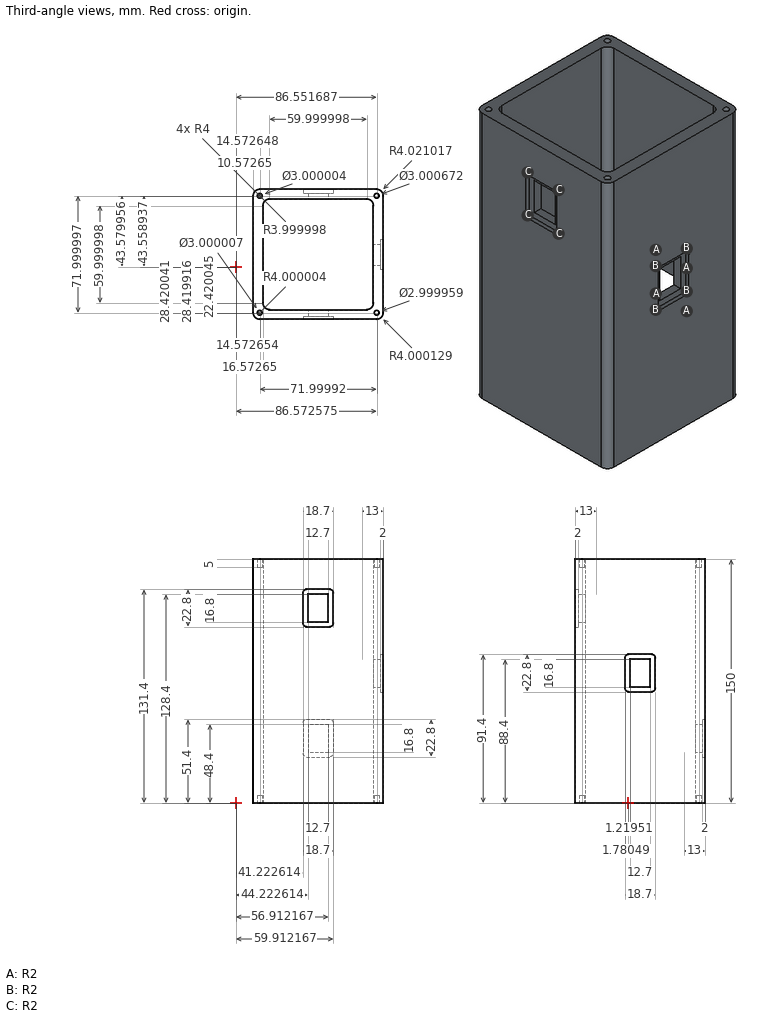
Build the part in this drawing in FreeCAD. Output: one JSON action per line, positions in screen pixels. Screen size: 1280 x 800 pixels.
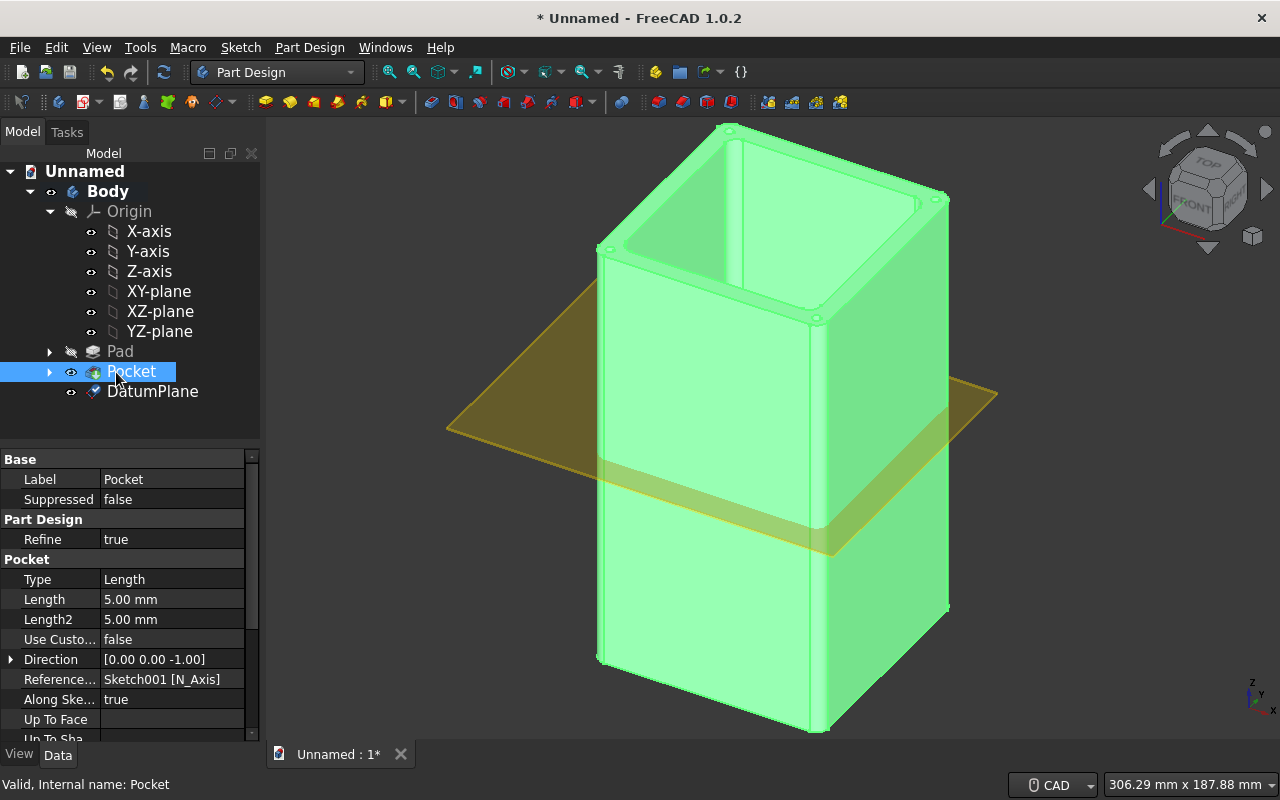
{"action": "left_click", "coordinate": [768, 102]}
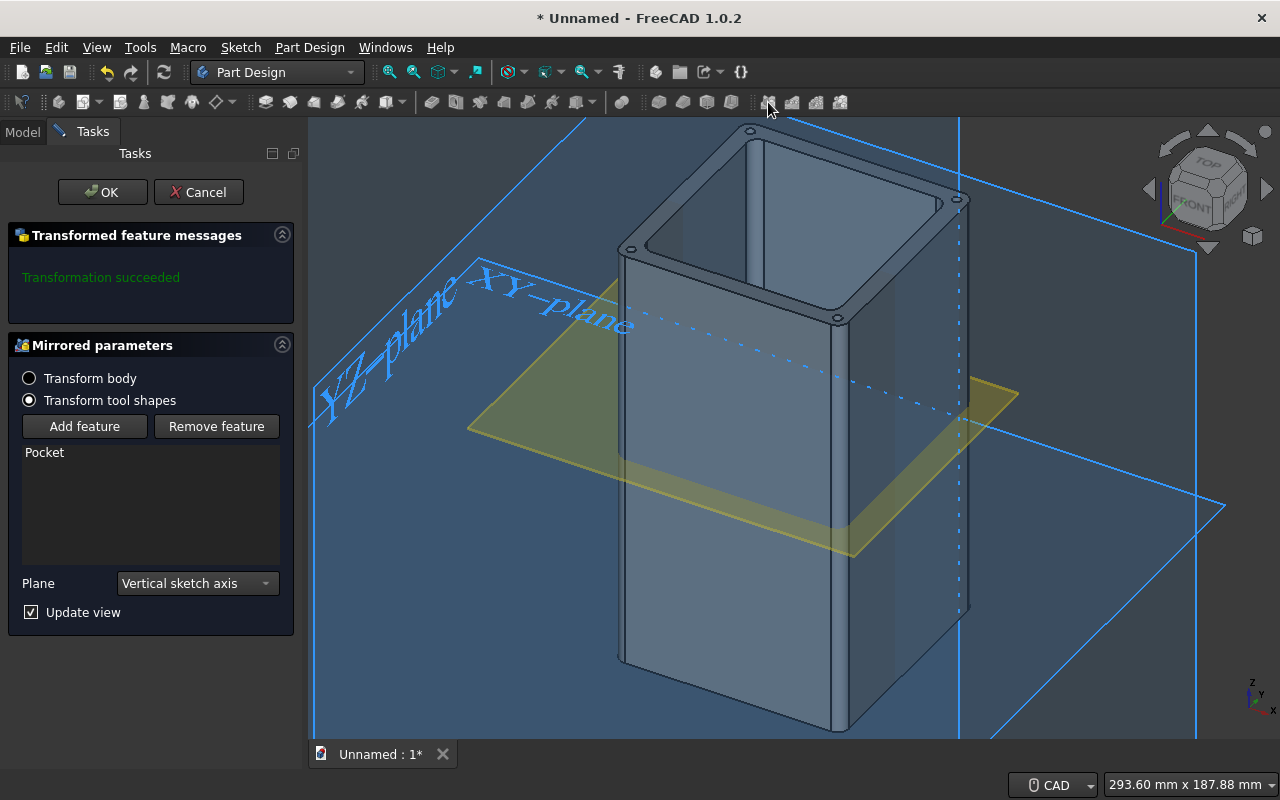
{"action": "left_click", "coordinate": [198, 584]}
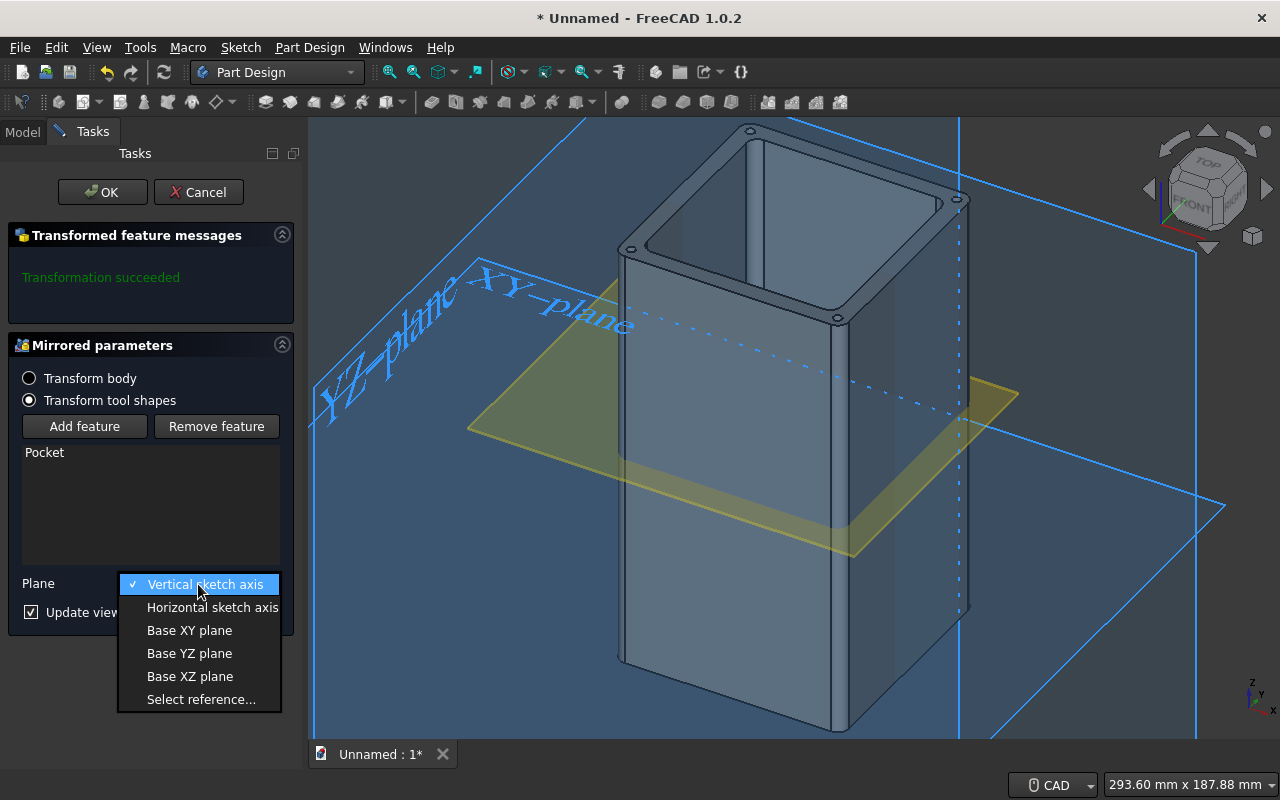
{"action": "left_click", "coordinate": [198, 700]}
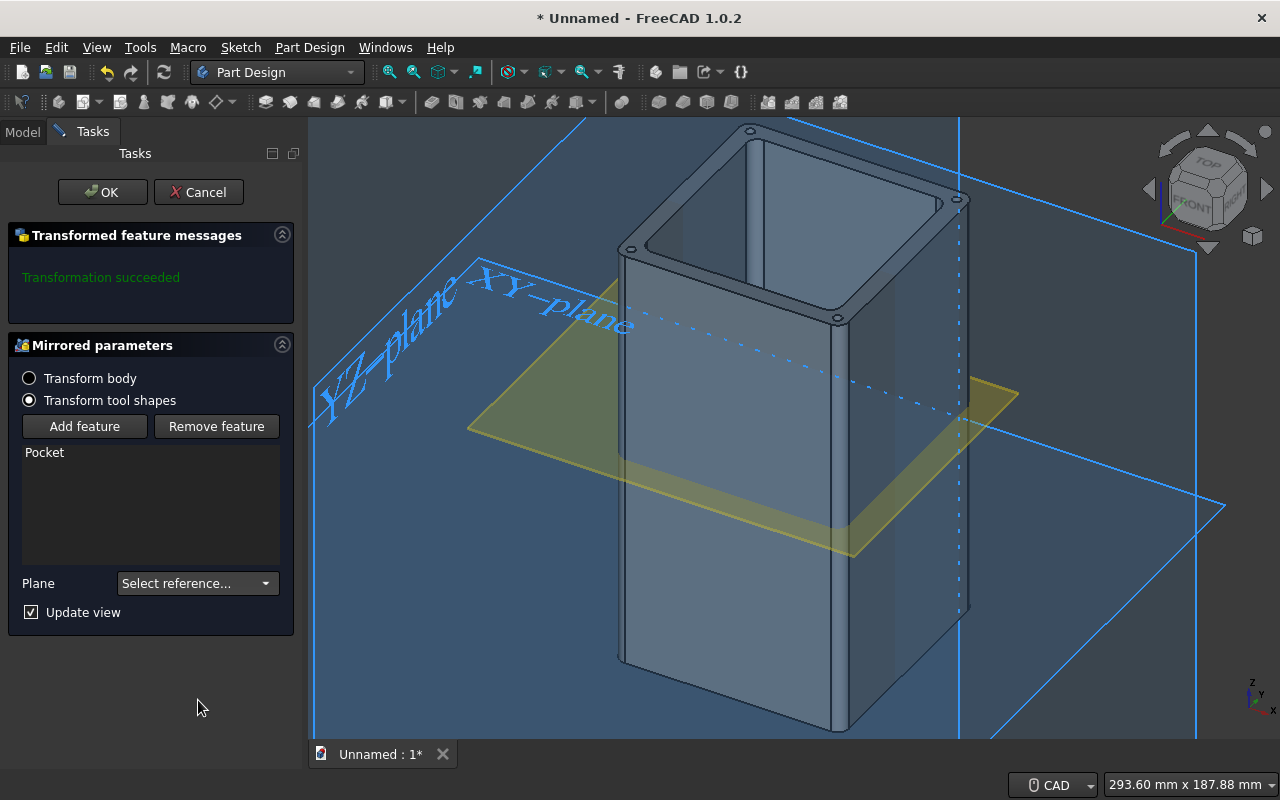
{"action": "left_click", "coordinate": [23, 131]}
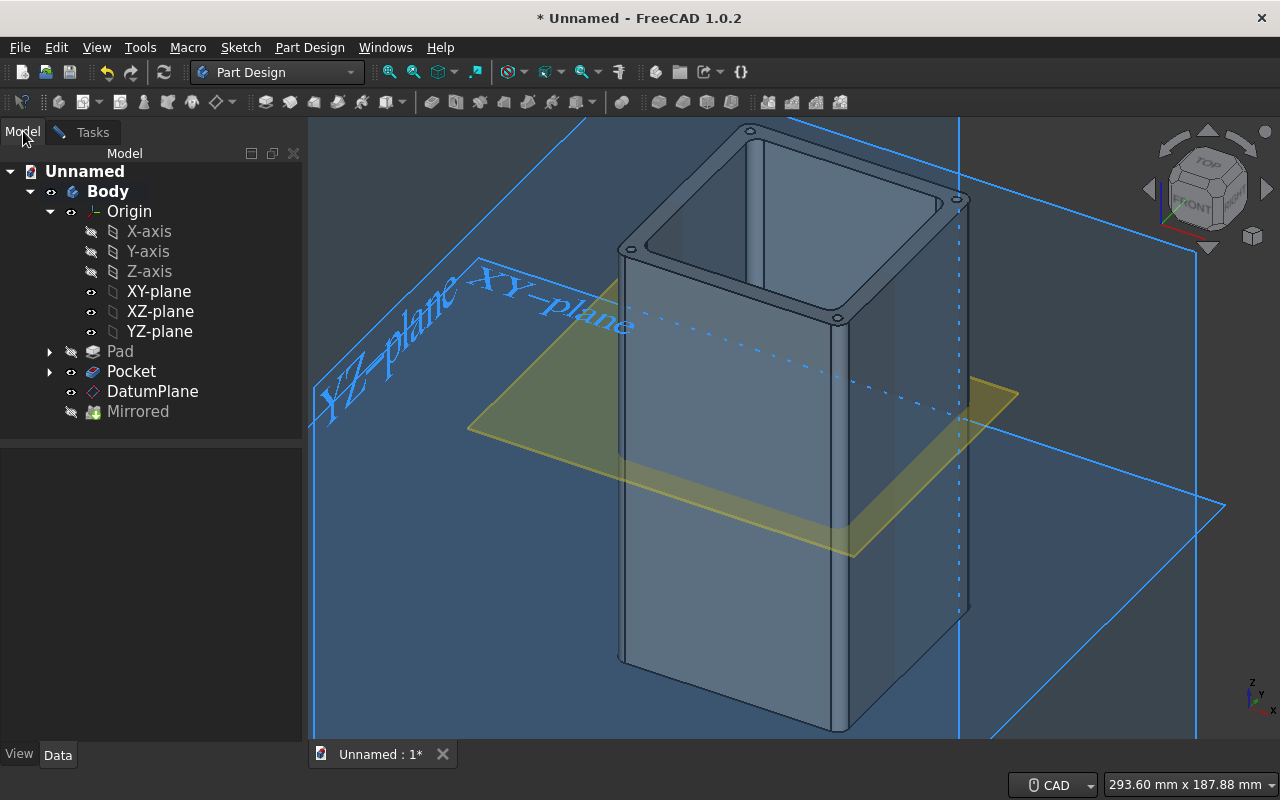
{"action": "left_click", "coordinate": [116, 392]}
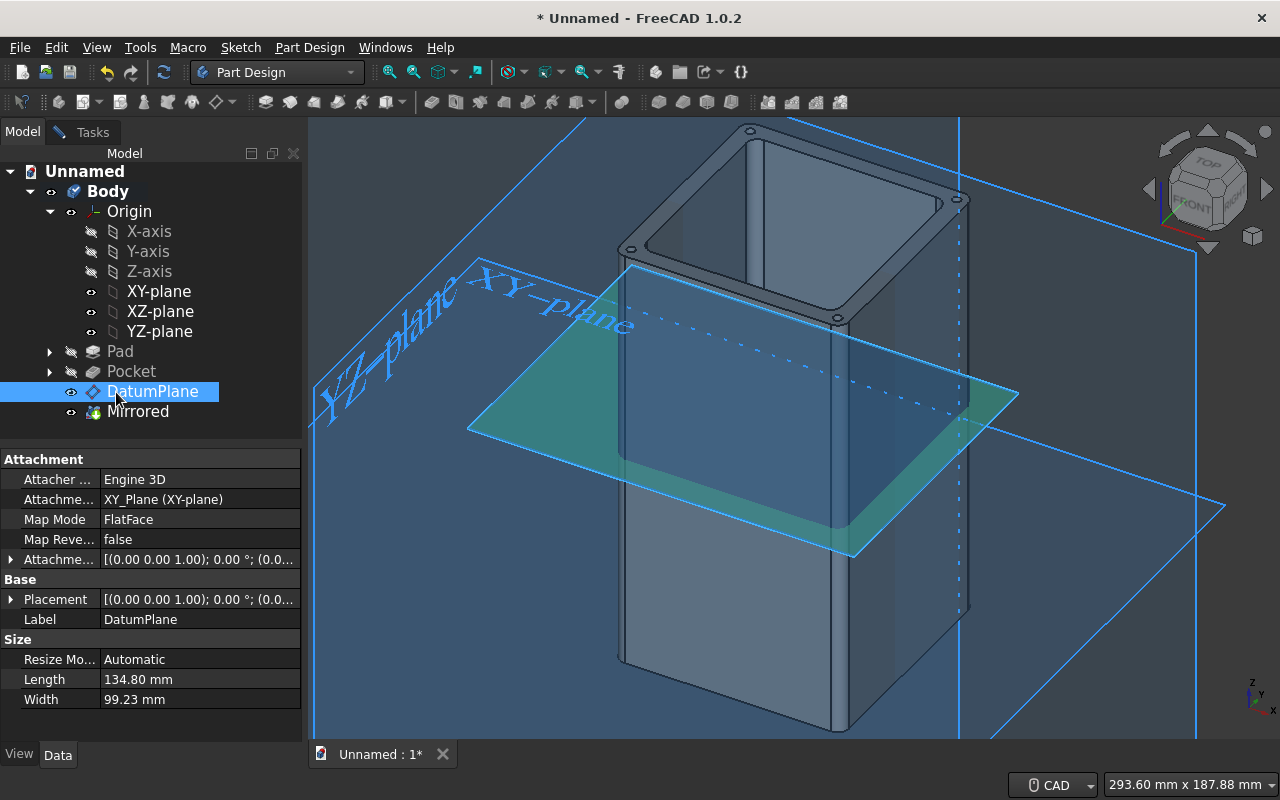
{"action": "left_click", "coordinate": [84, 131]}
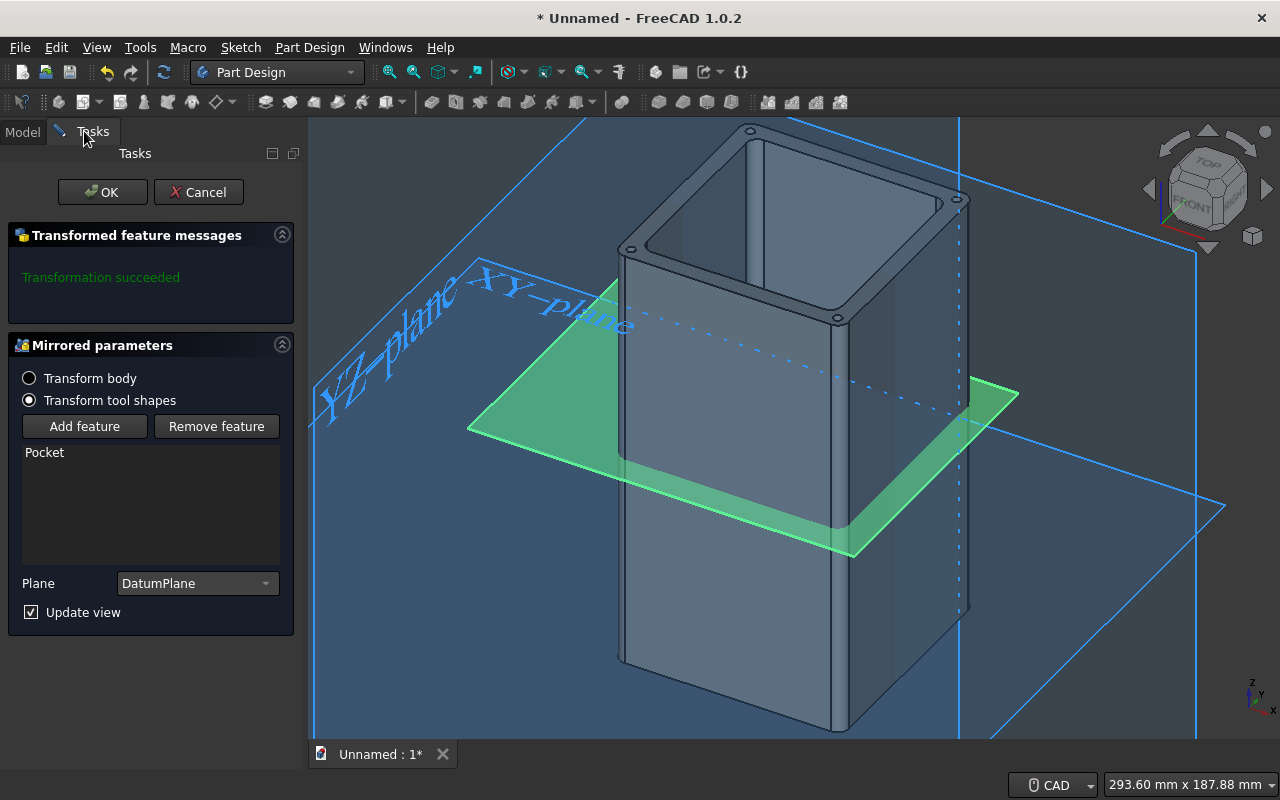
{"action": "left_click", "coordinate": [103, 192]}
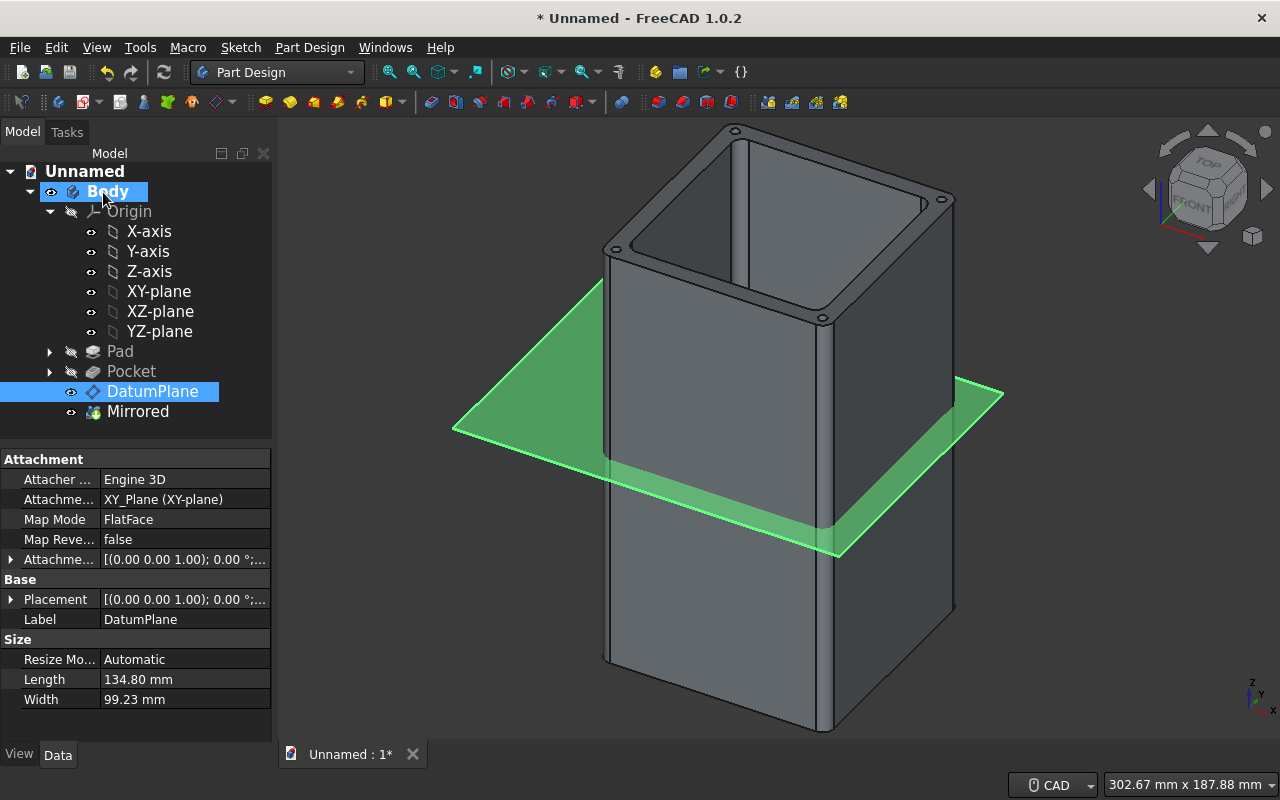
{"action": "left_click", "coordinate": [116, 392]}
{"action": "key", "text": "space"}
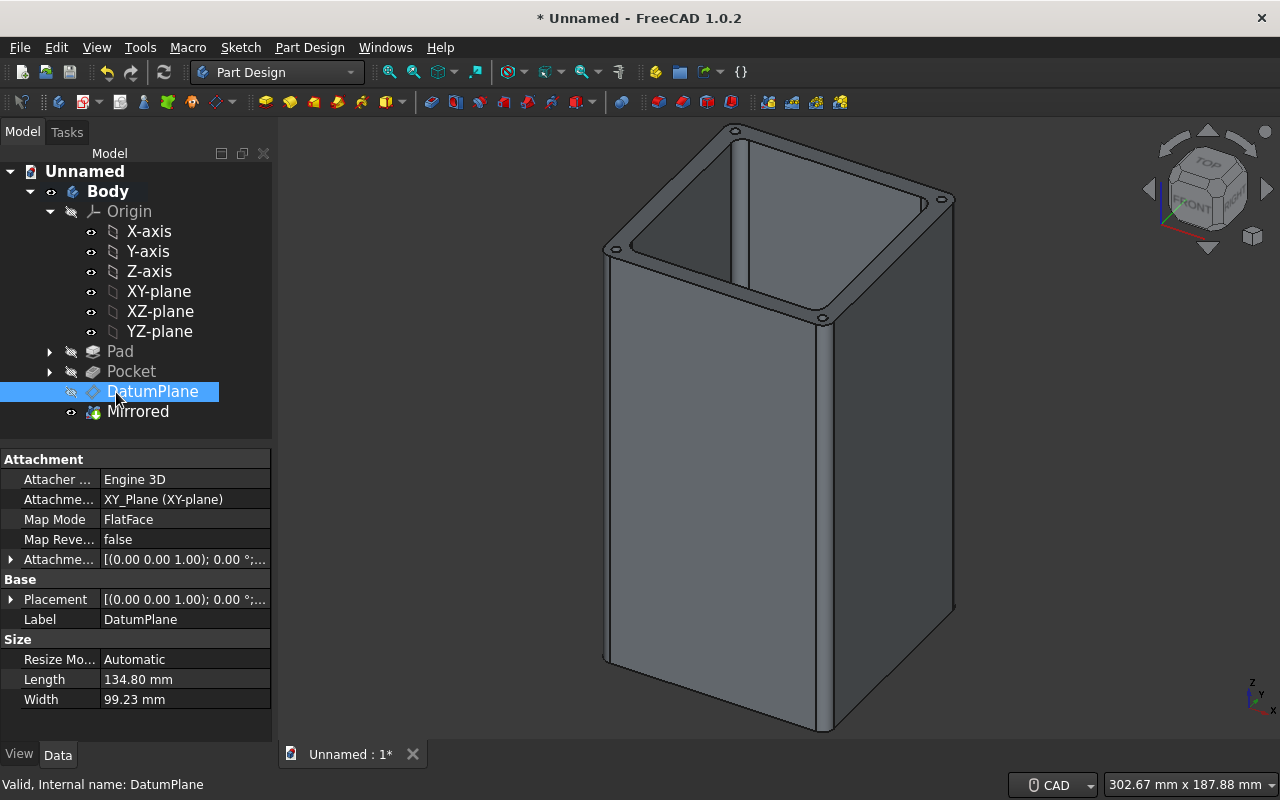
{"action": "key", "text": "4"}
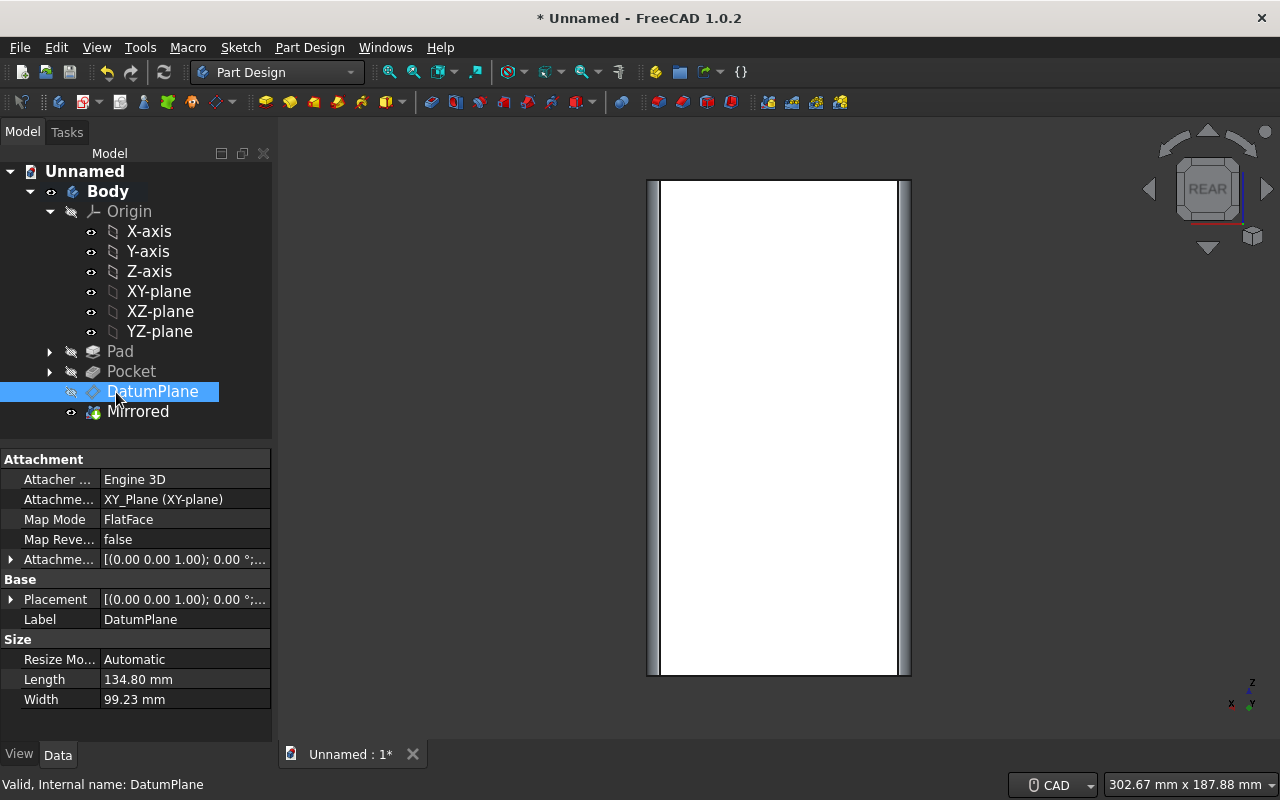
{"action": "left_click", "coordinate": [779, 356]}